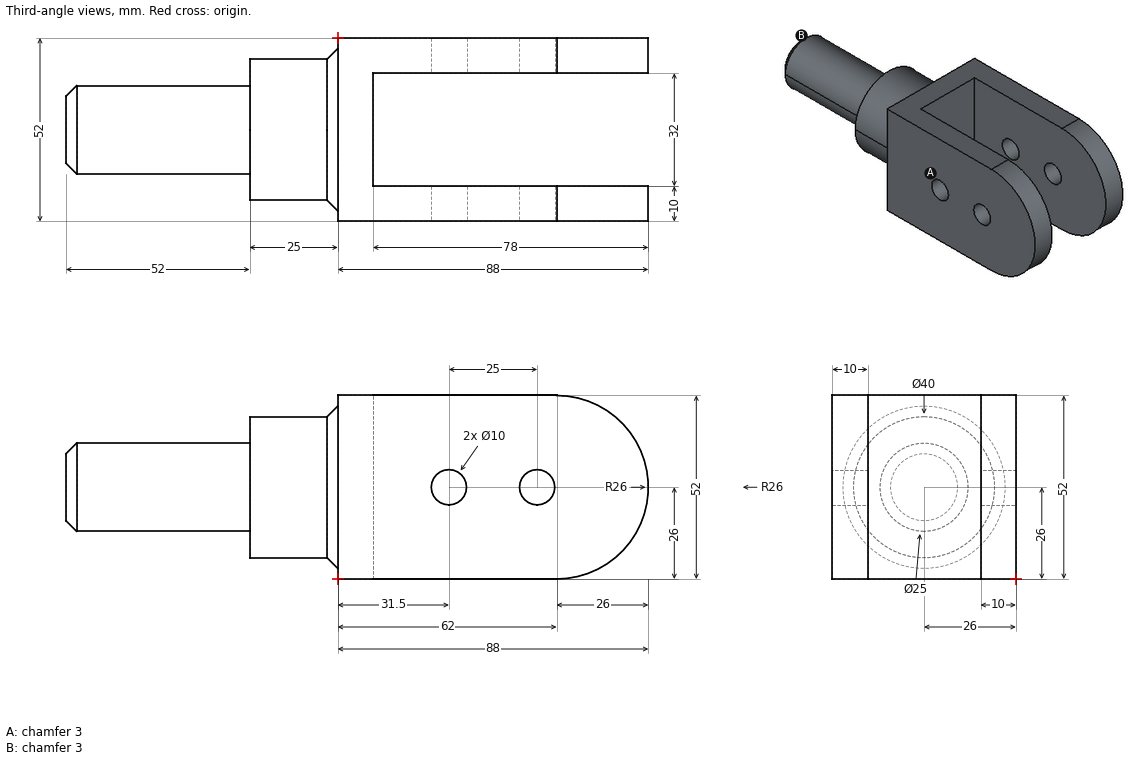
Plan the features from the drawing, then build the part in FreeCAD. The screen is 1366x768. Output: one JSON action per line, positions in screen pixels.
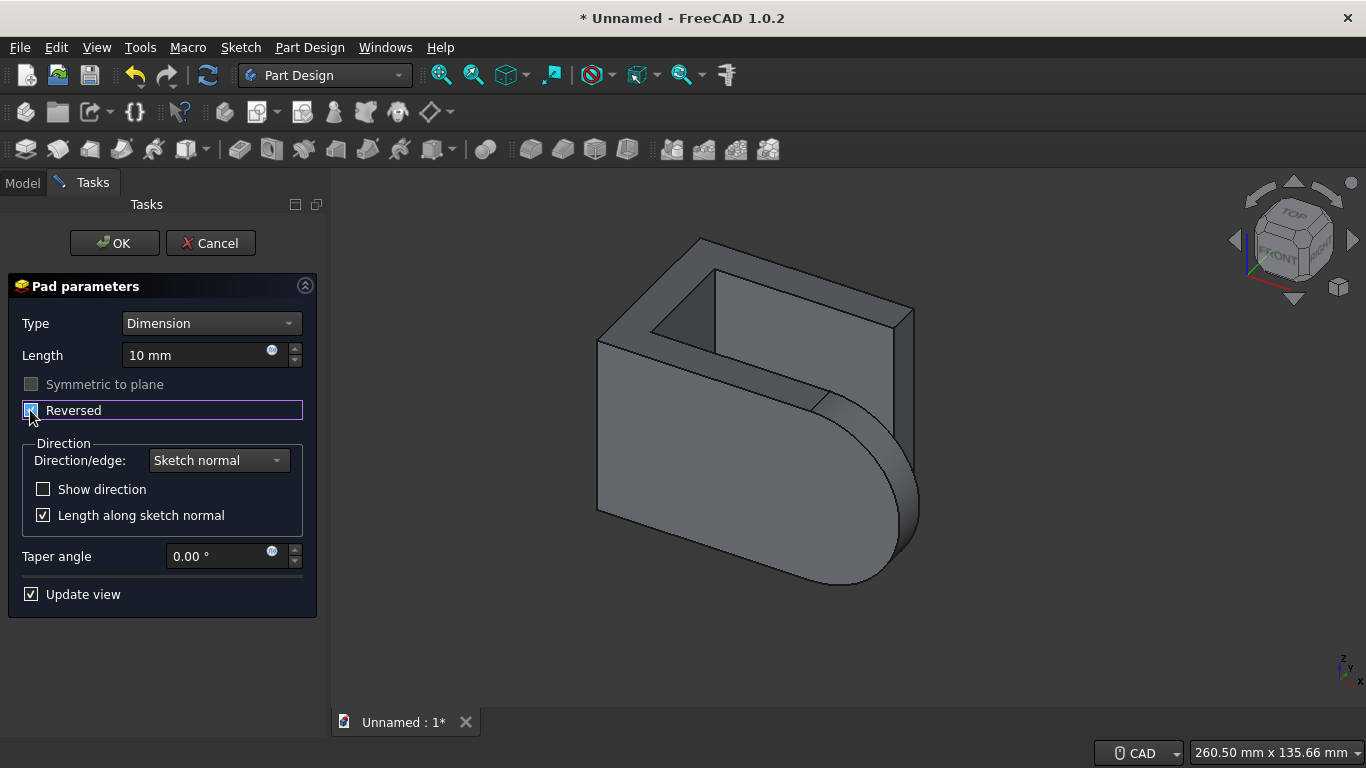
{"action": "left_click", "coordinate": [115, 243]}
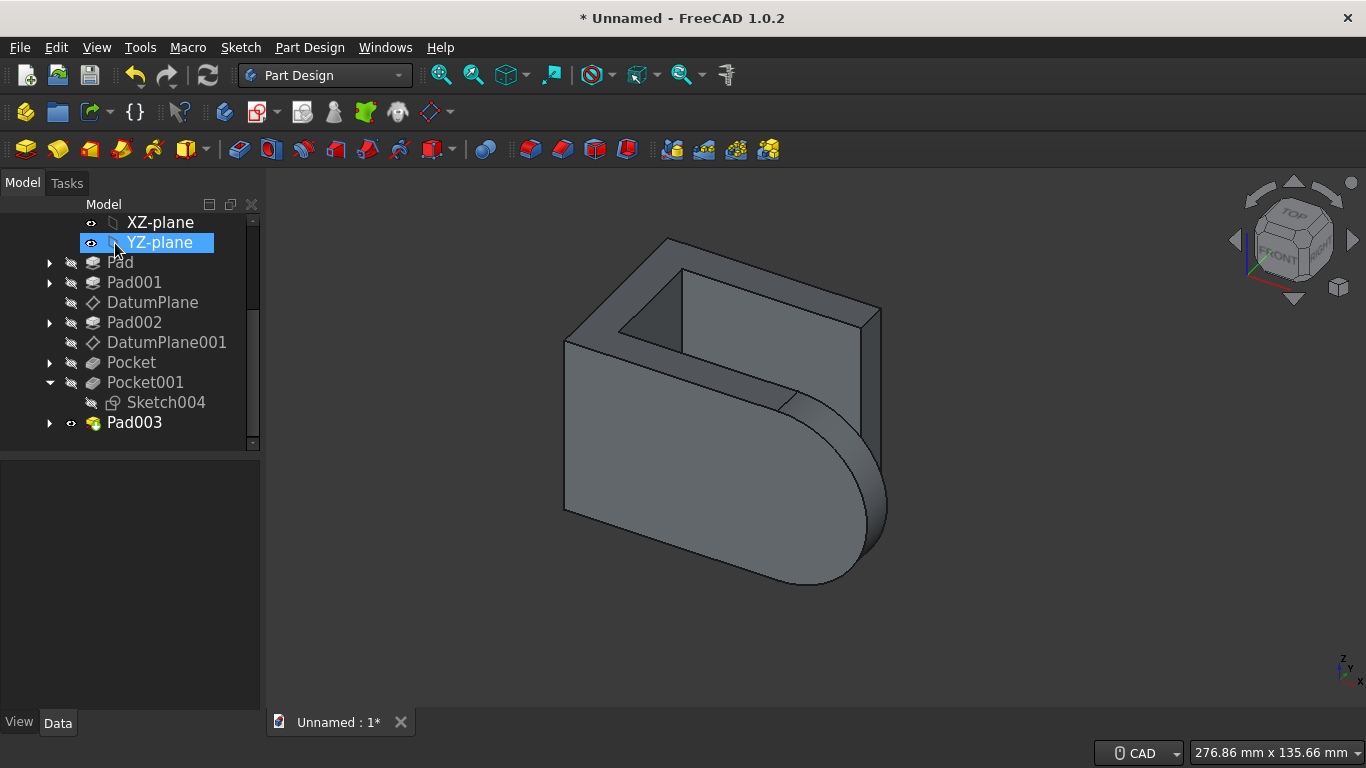
{"action": "scroll", "coordinate": [160, 318], "scroll_direction": "down", "scroll_amount": 3}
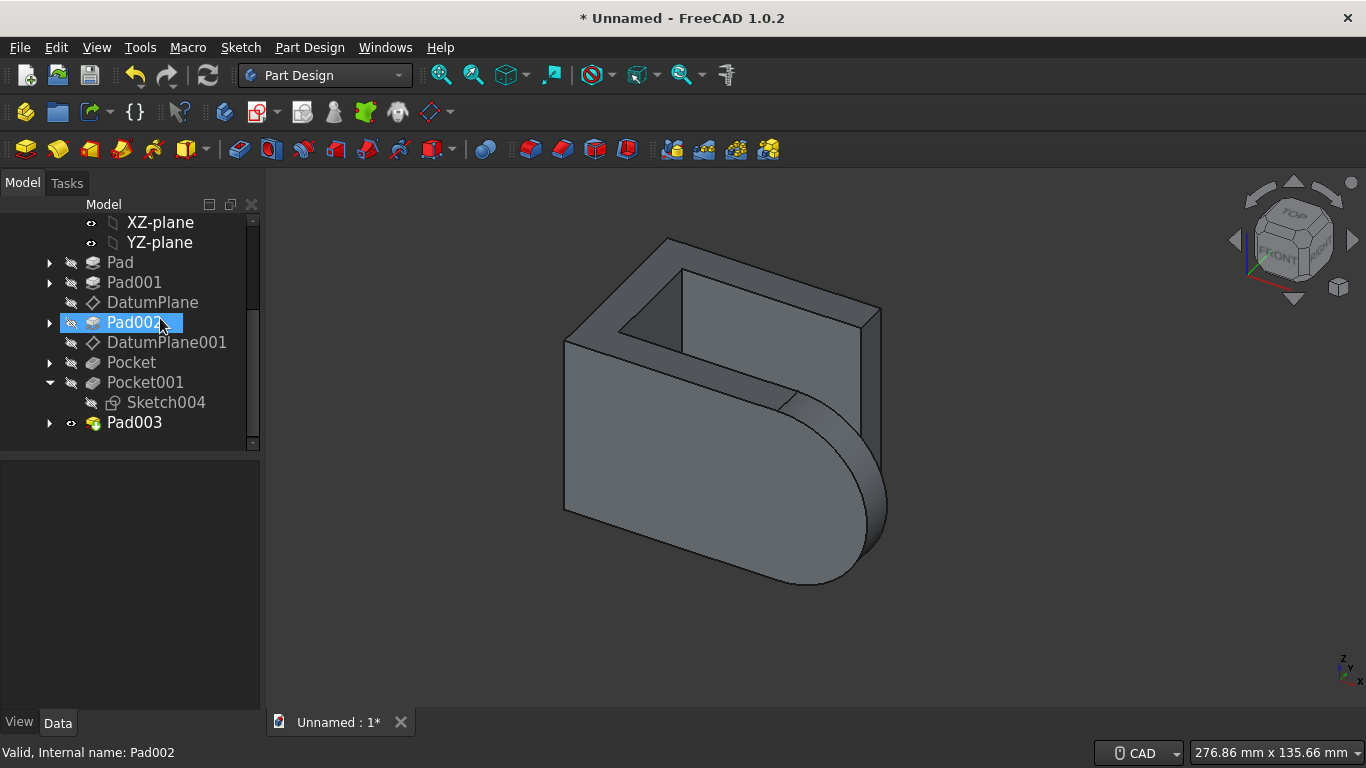
{"action": "scroll", "coordinate": [160, 318], "scroll_direction": "up", "scroll_amount": 15}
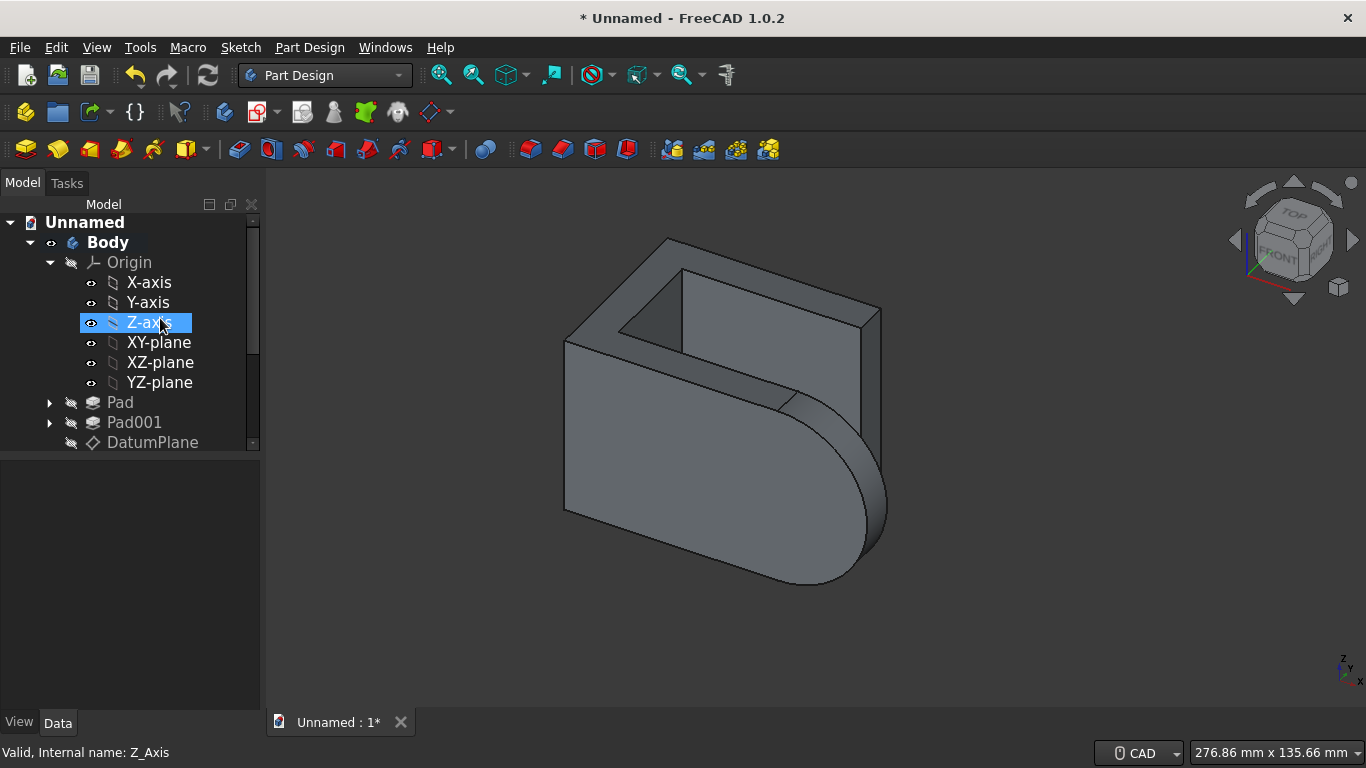
{"action": "left_click", "coordinate": [136, 363]}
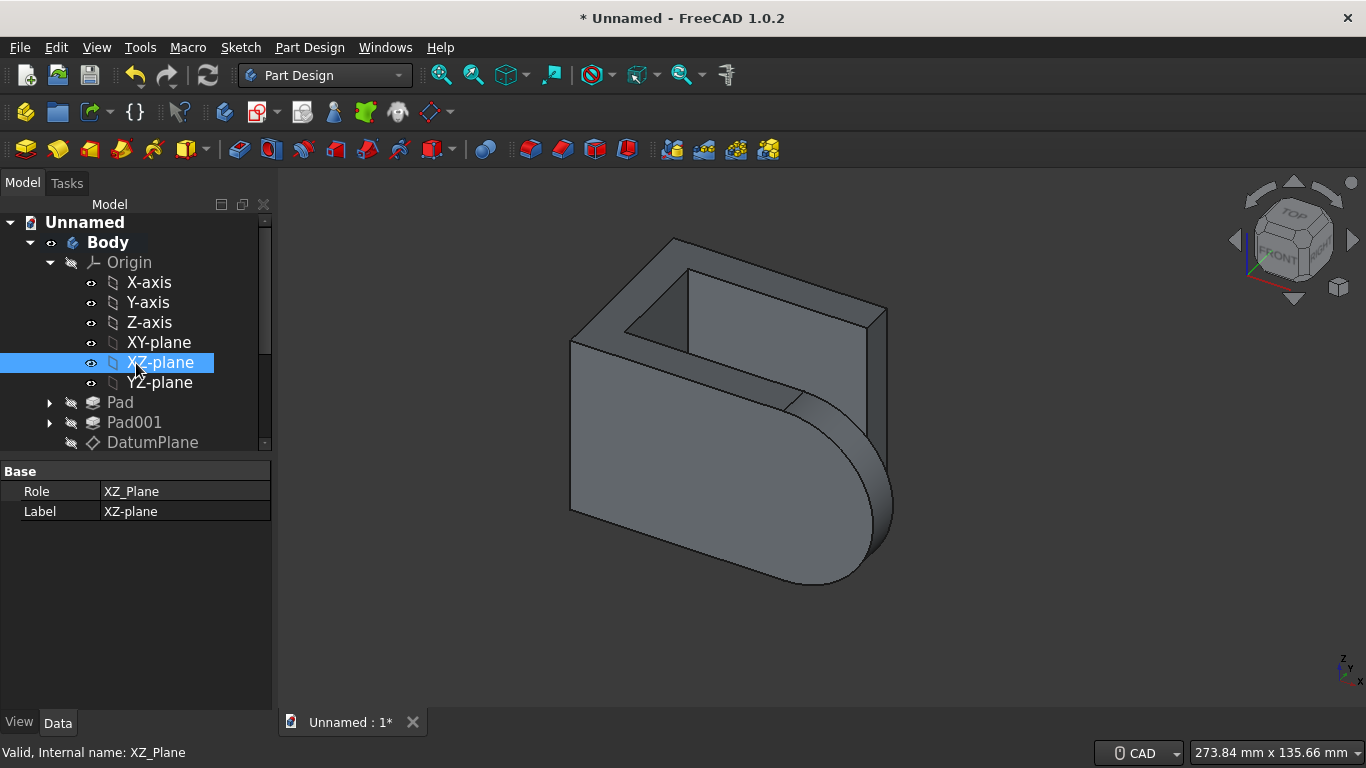
{"action": "left_click", "coordinate": [430, 112]}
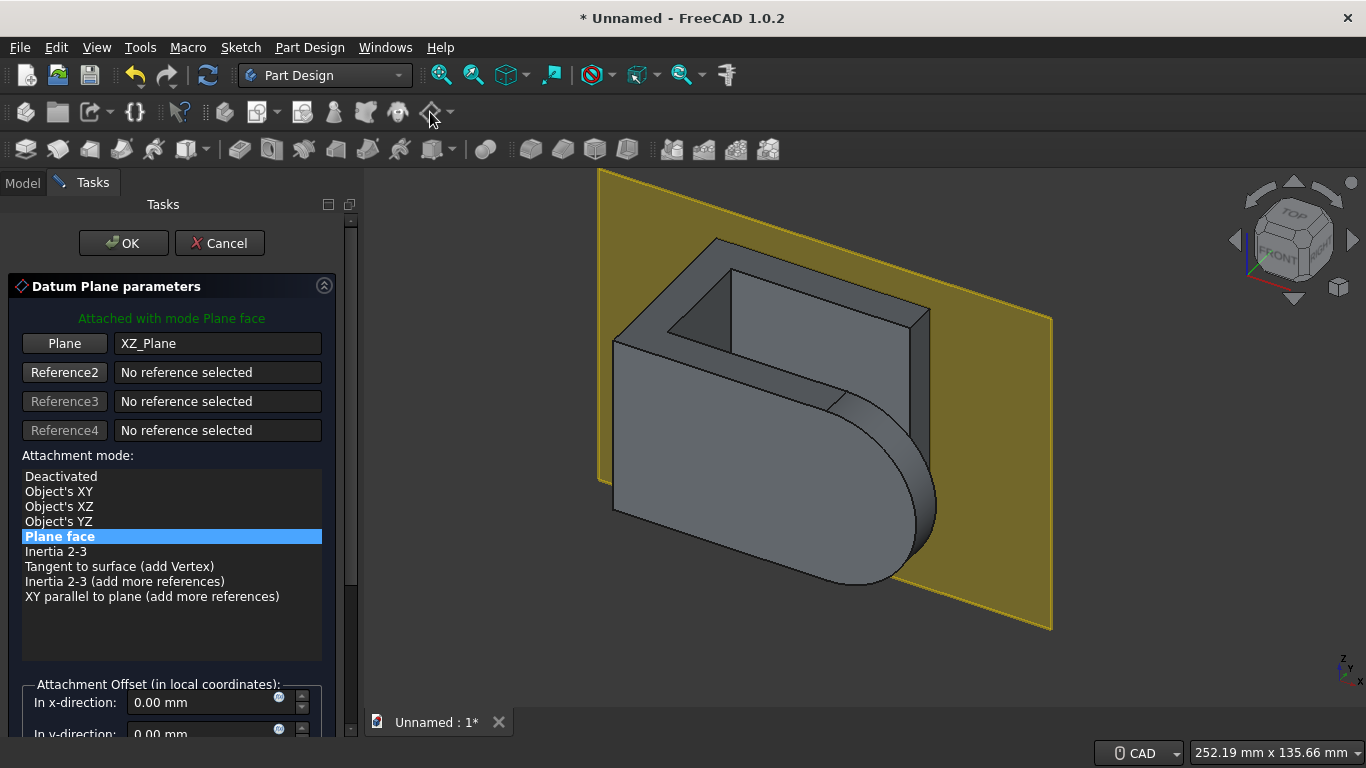
{"action": "scroll", "coordinate": [351, 475], "scroll_direction": "down", "scroll_amount": 2}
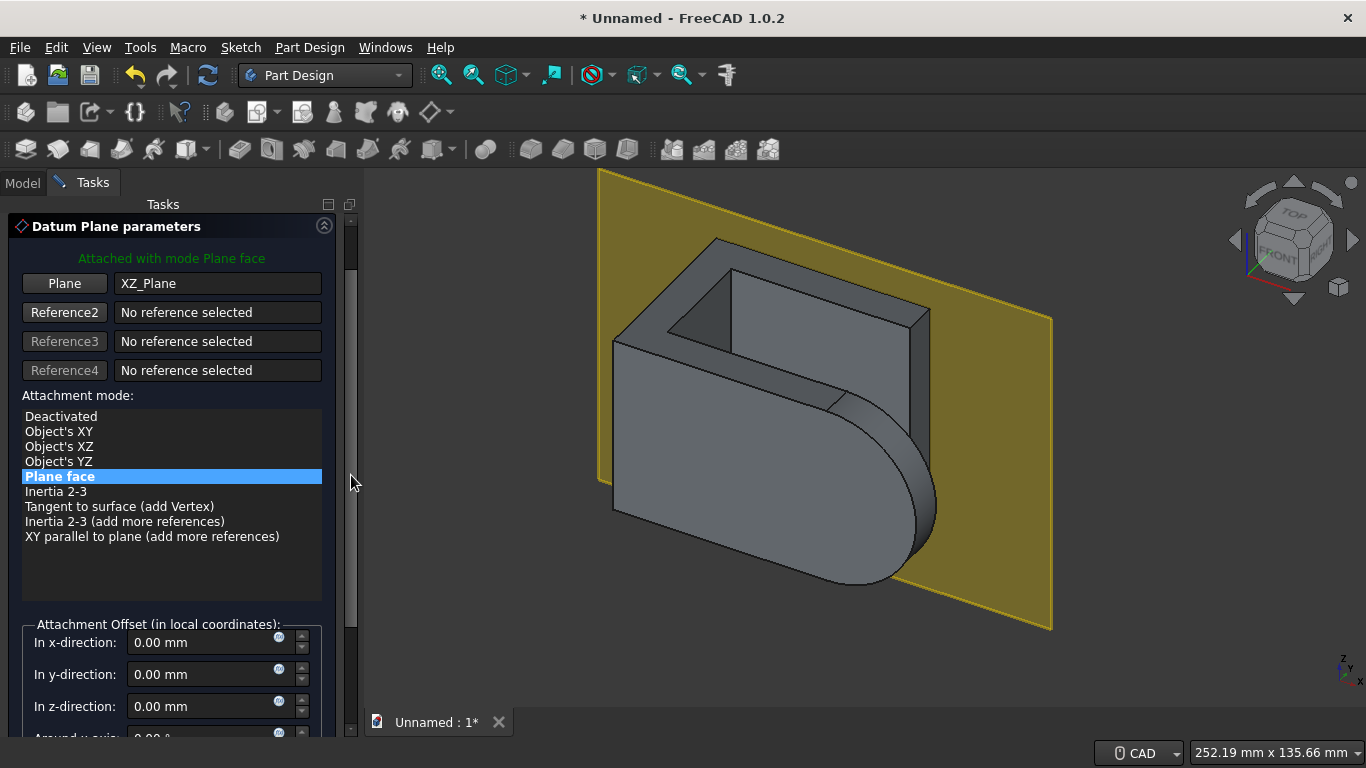
{"action": "triple_click", "coordinate": [210, 646]}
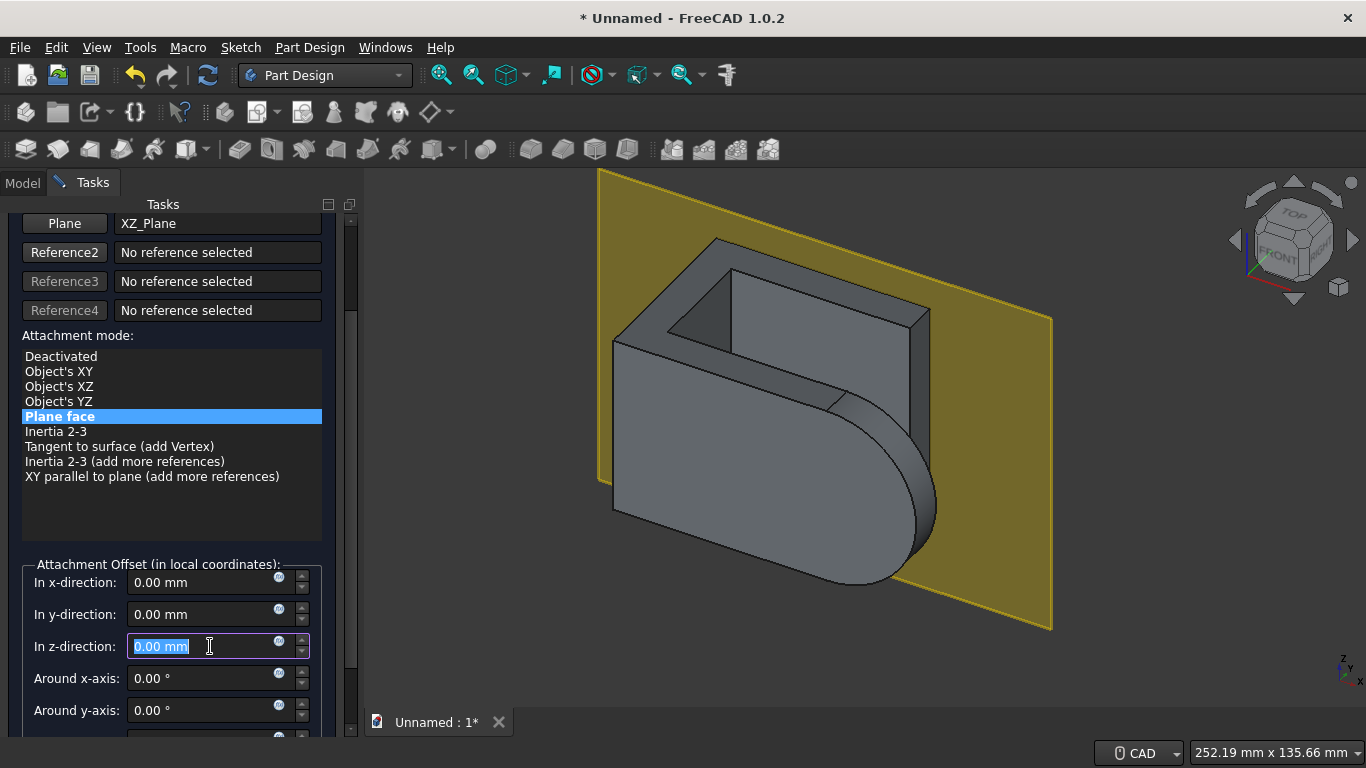
{"action": "type", "text": "10"}
{"action": "key", "text": "Tab"}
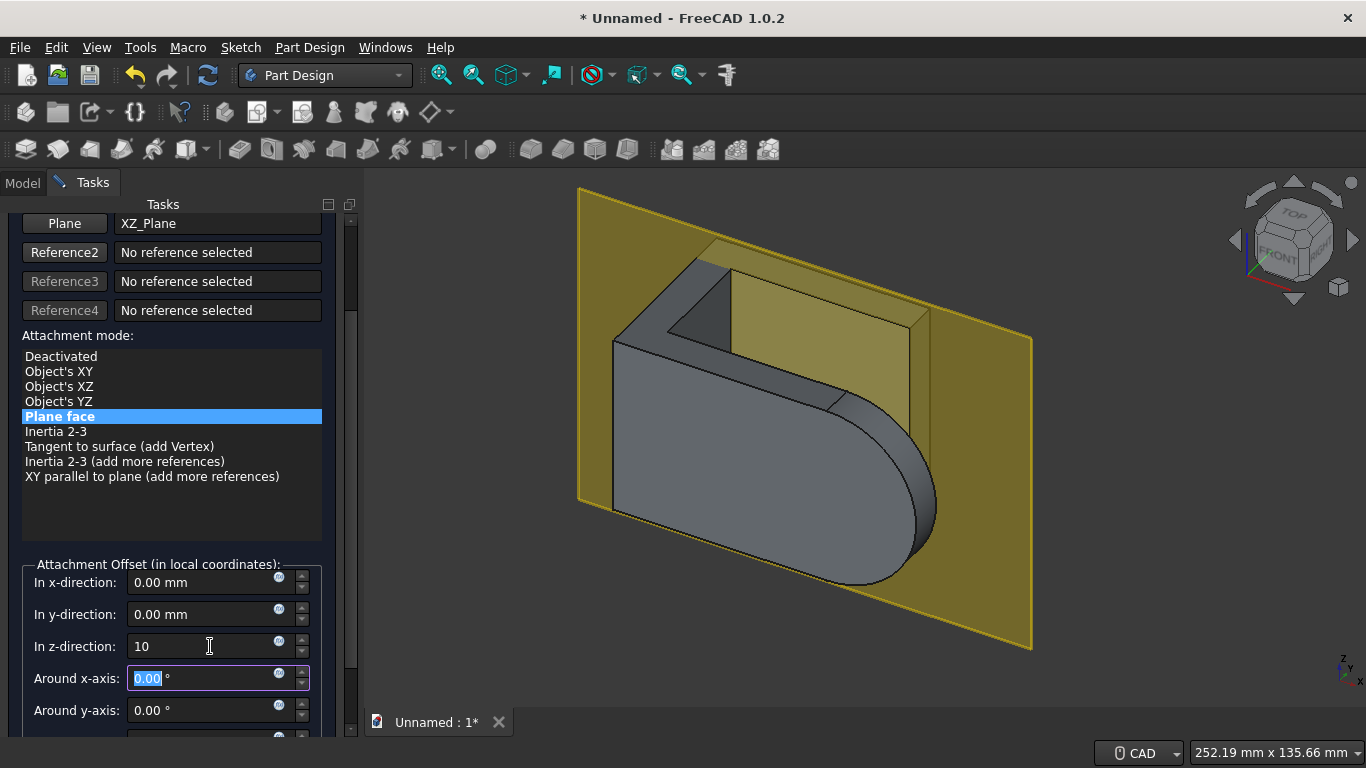
{"action": "scroll", "coordinate": [351, 475], "scroll_direction": "up", "scroll_amount": 3}